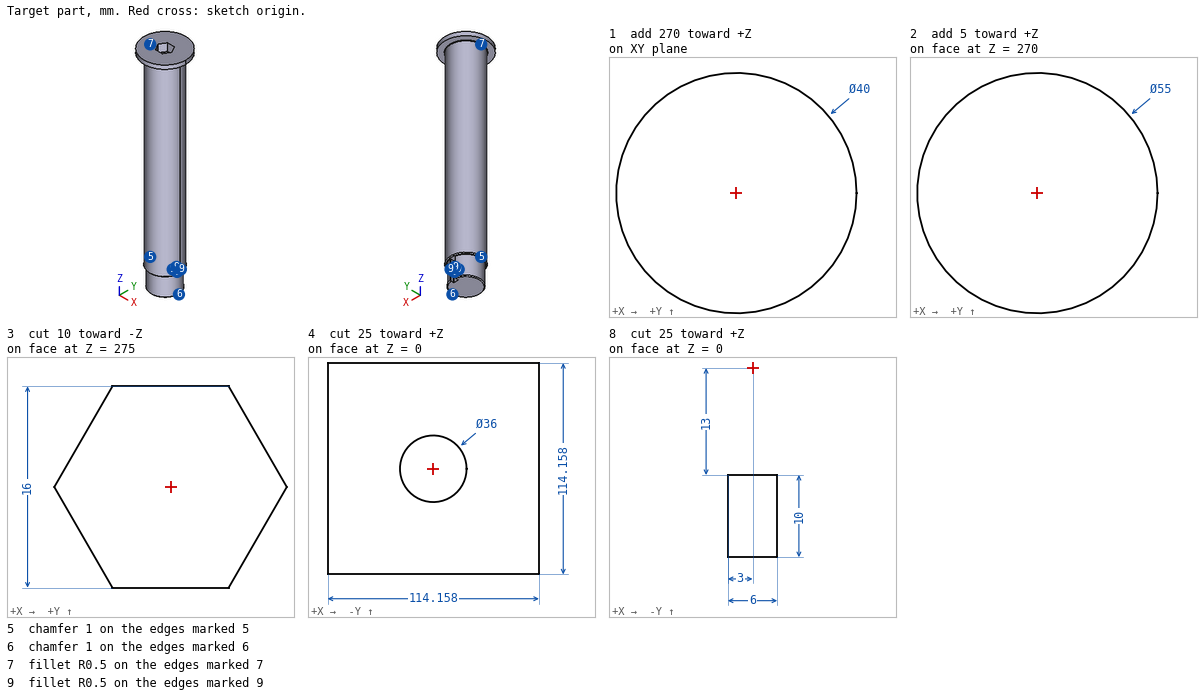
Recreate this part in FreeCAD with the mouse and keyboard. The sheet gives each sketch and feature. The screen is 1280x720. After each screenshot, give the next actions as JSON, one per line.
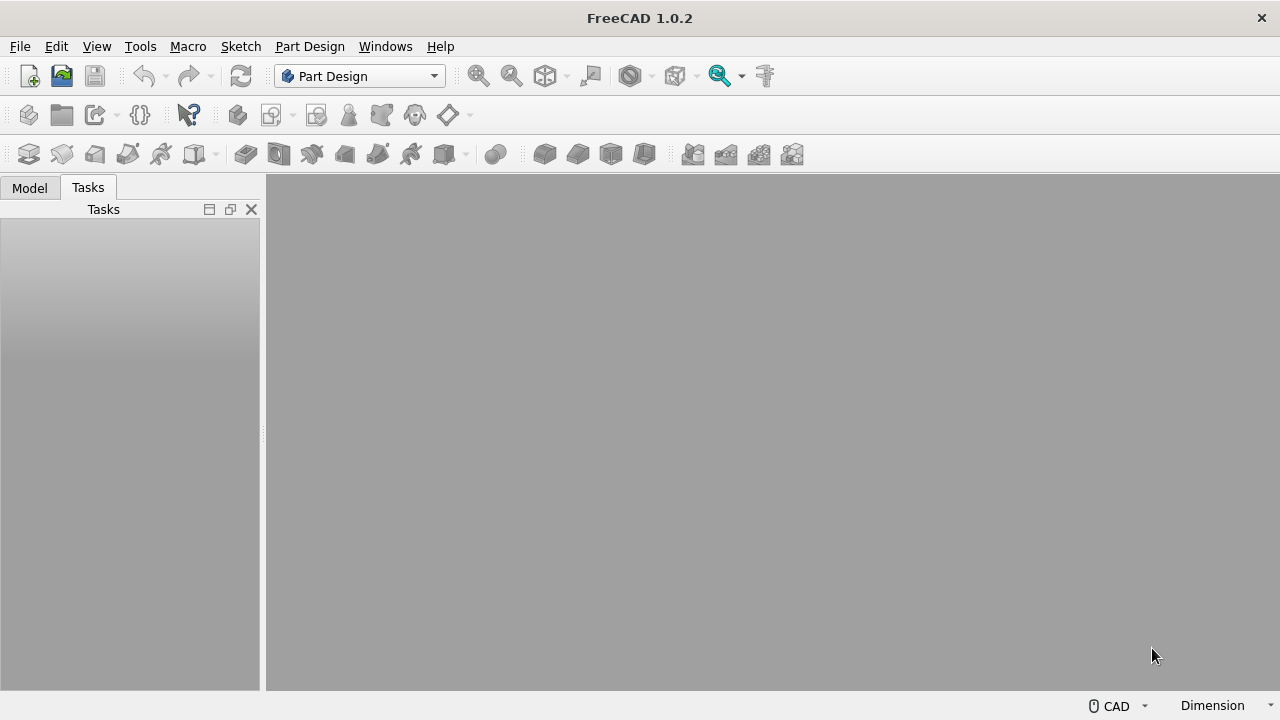
{"action": "left_click", "coordinate": [29, 76]}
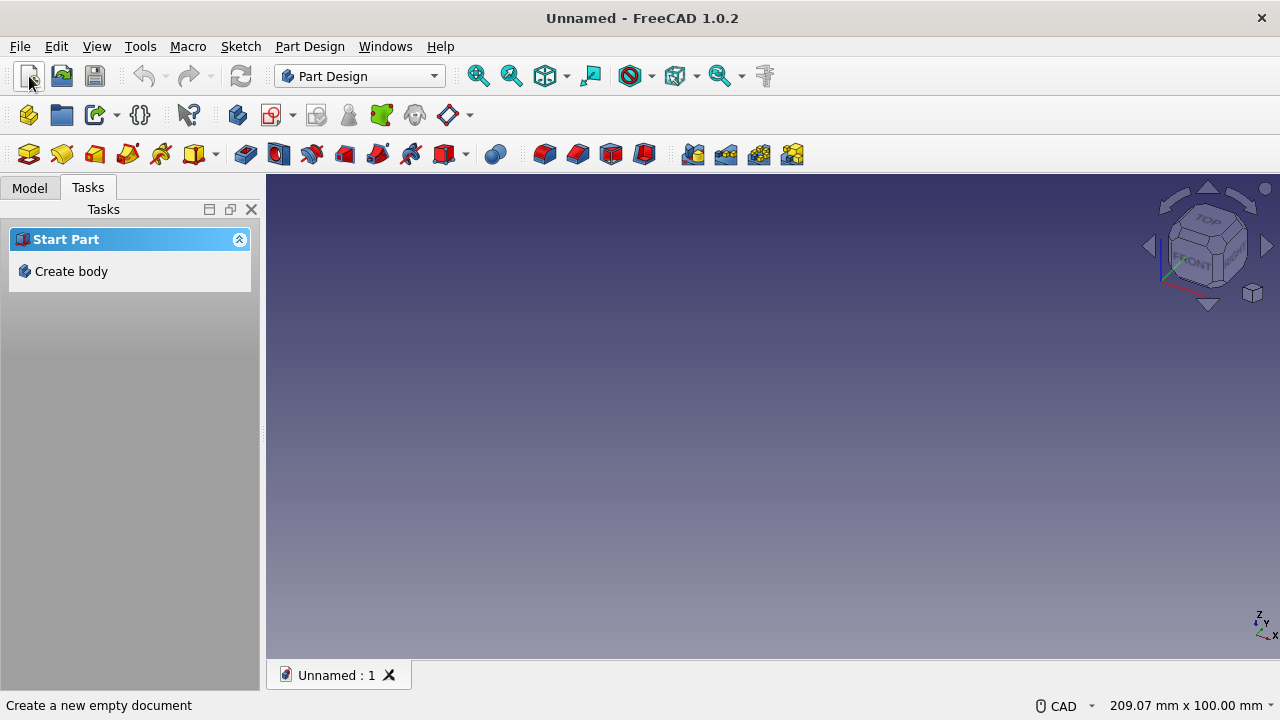
{"action": "left_click", "coordinate": [270, 116]}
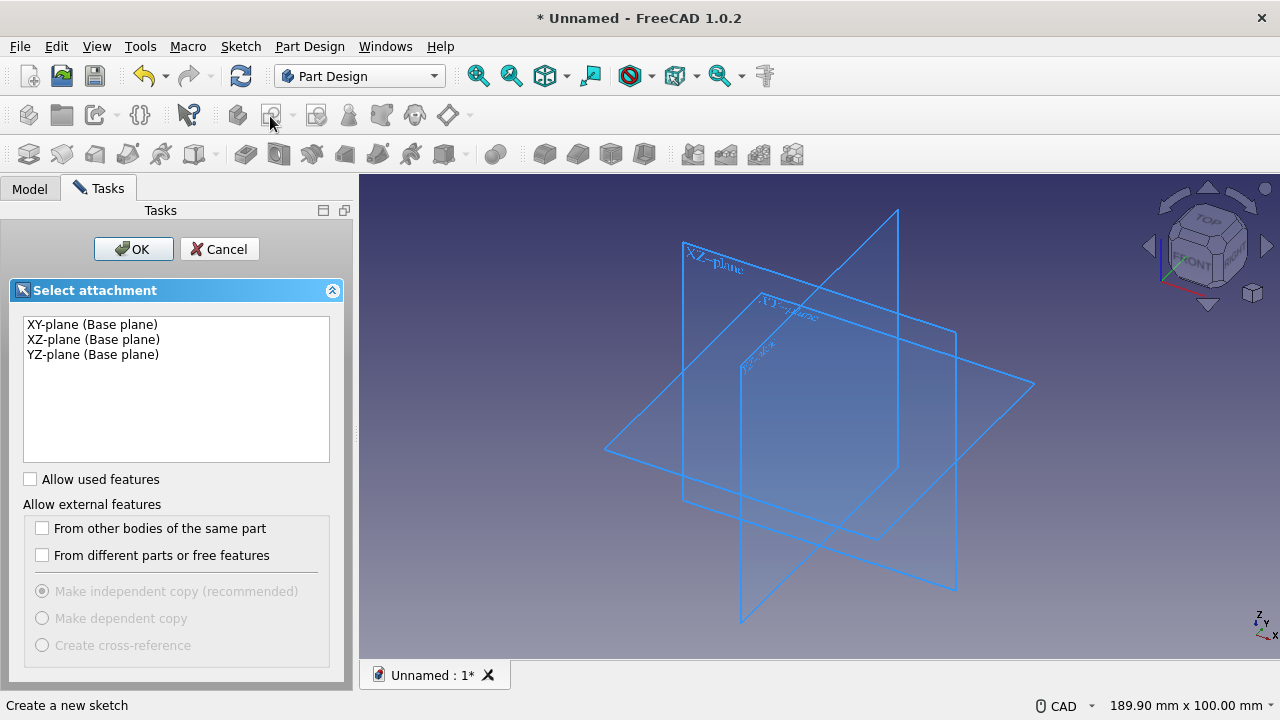
{"action": "left_click", "coordinate": [84, 324]}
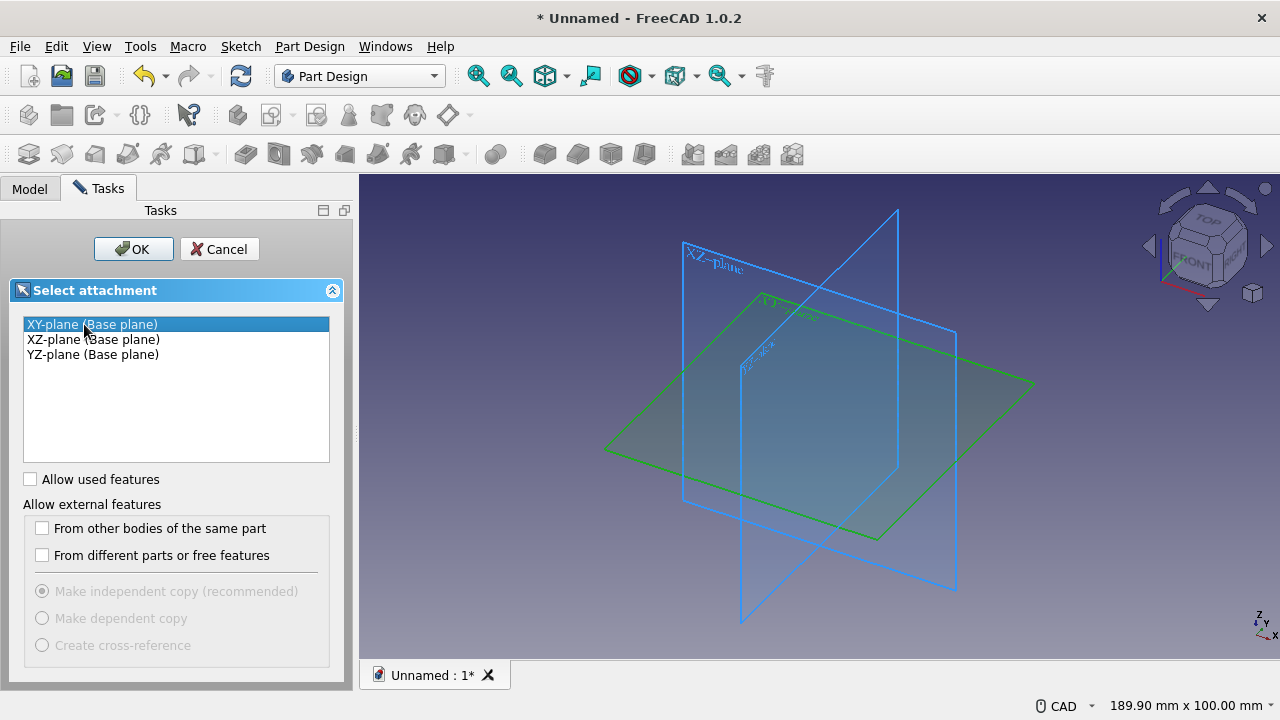
{"action": "left_click", "coordinate": [134, 249]}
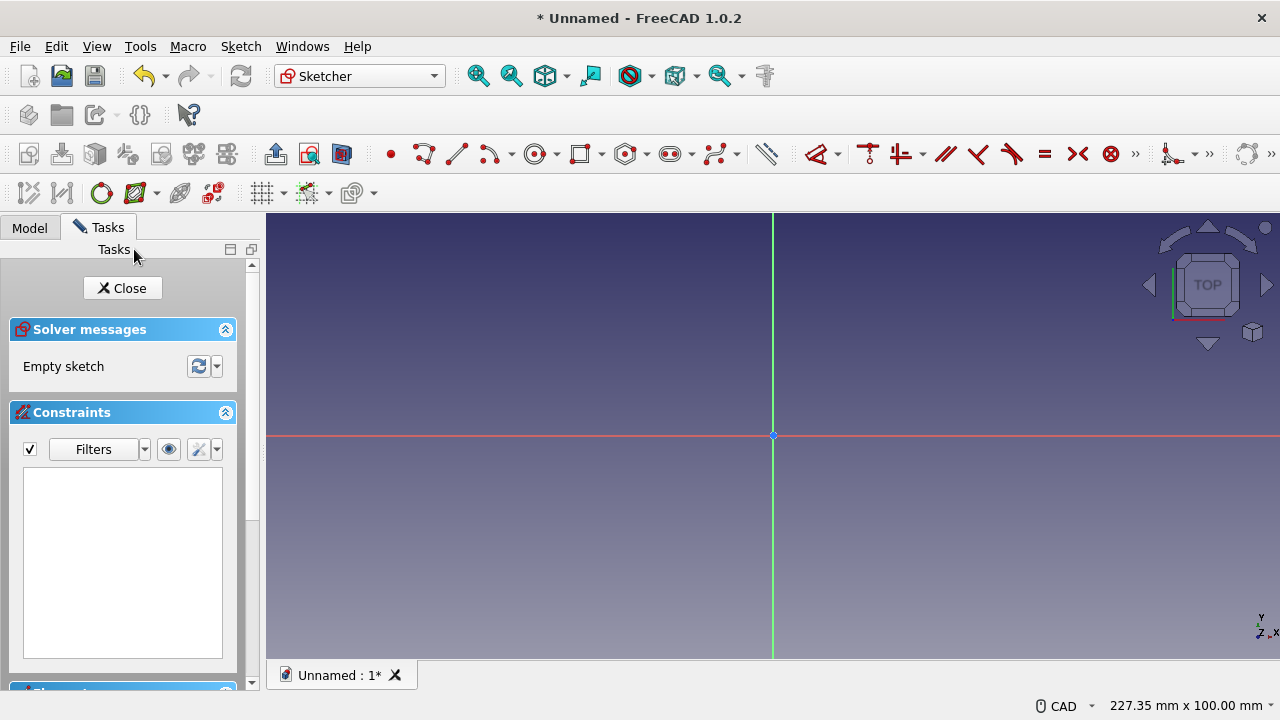
{"action": "scroll", "coordinate": [912, 436], "scroll_direction": "up", "scroll_amount": 2}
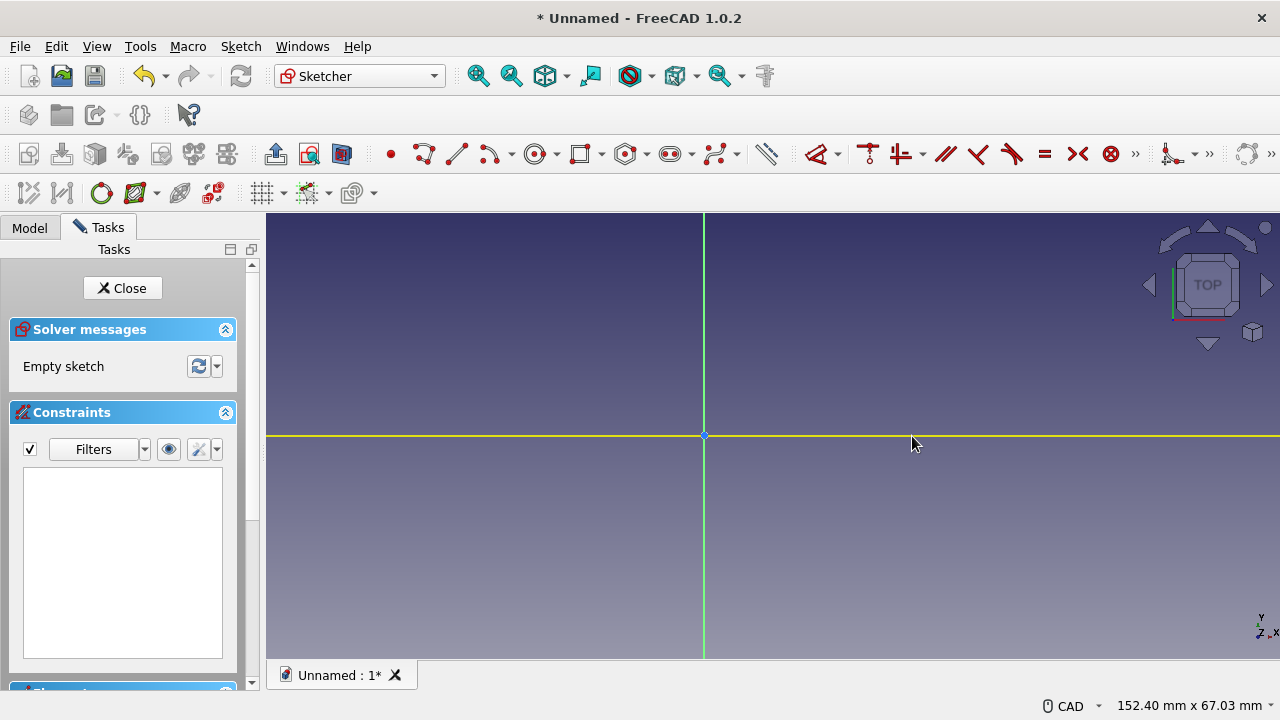
{"action": "left_click", "coordinate": [534, 154]}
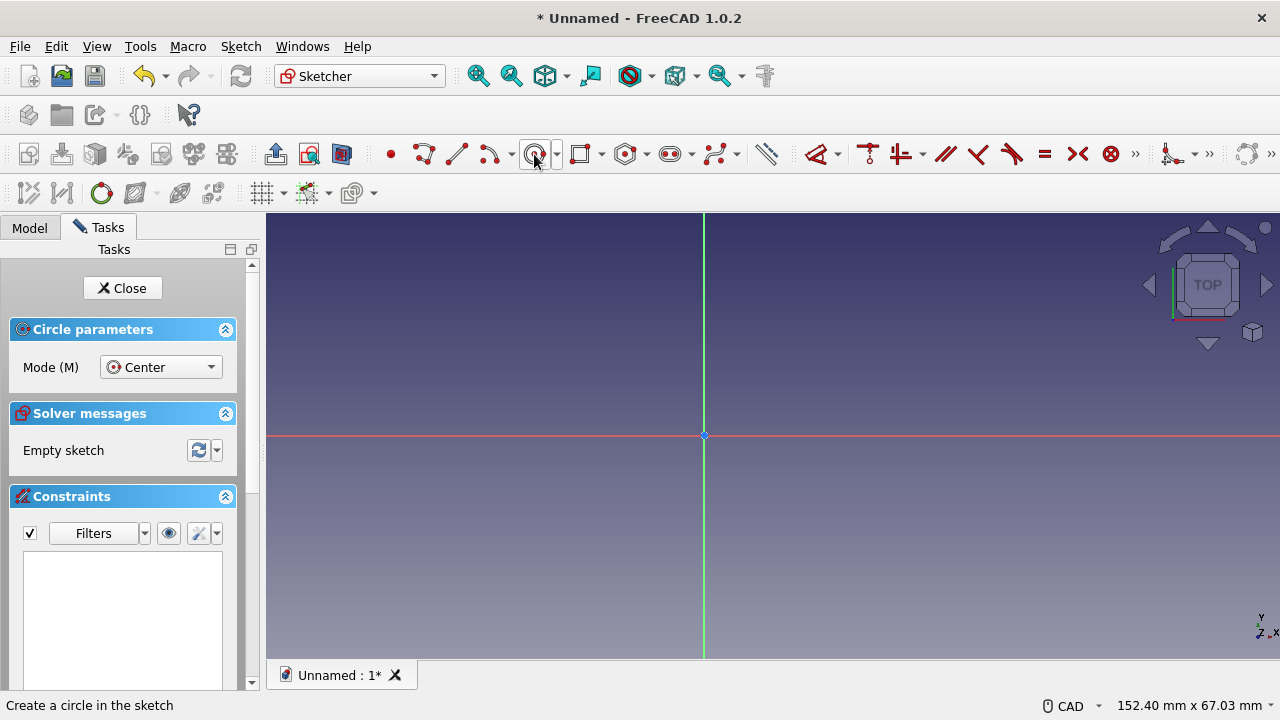
{"action": "left_click", "coordinate": [704, 436]}
{"action": "mouse_move", "coordinate": [798, 342]}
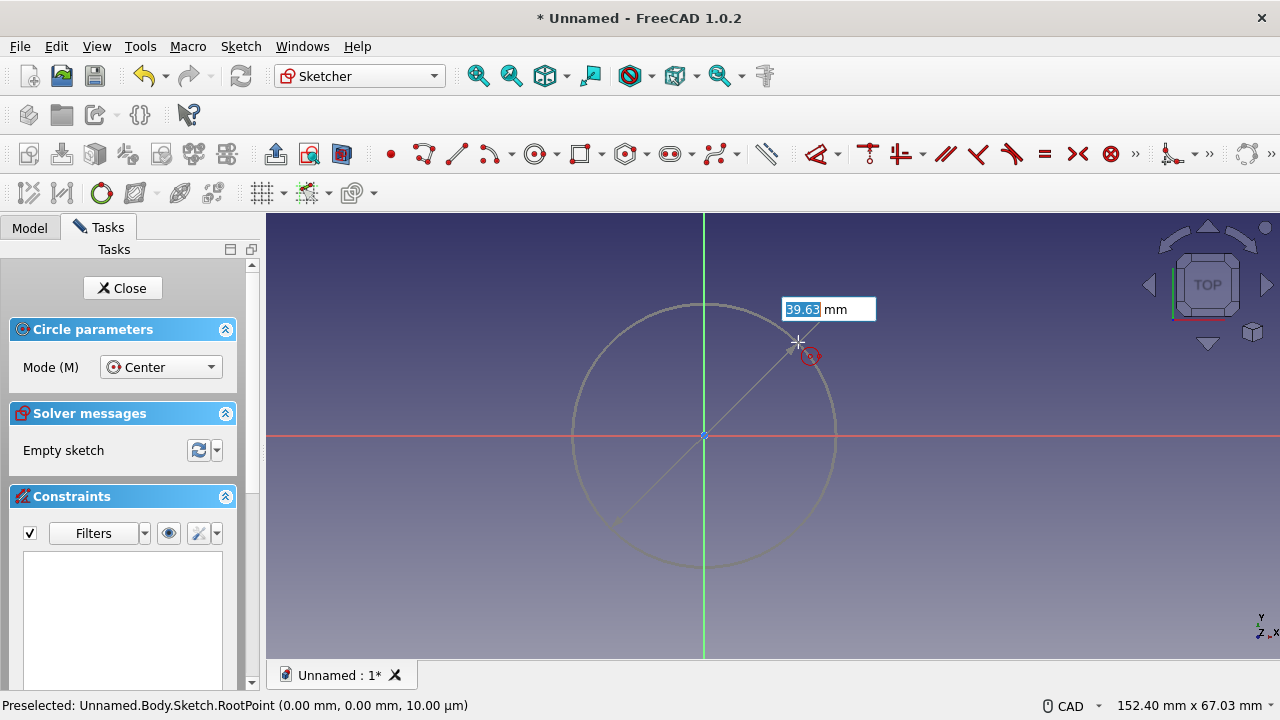
{"action": "type", "text": "40"}
{"action": "key", "text": "Return"}
{"action": "key", "text": "Escape"}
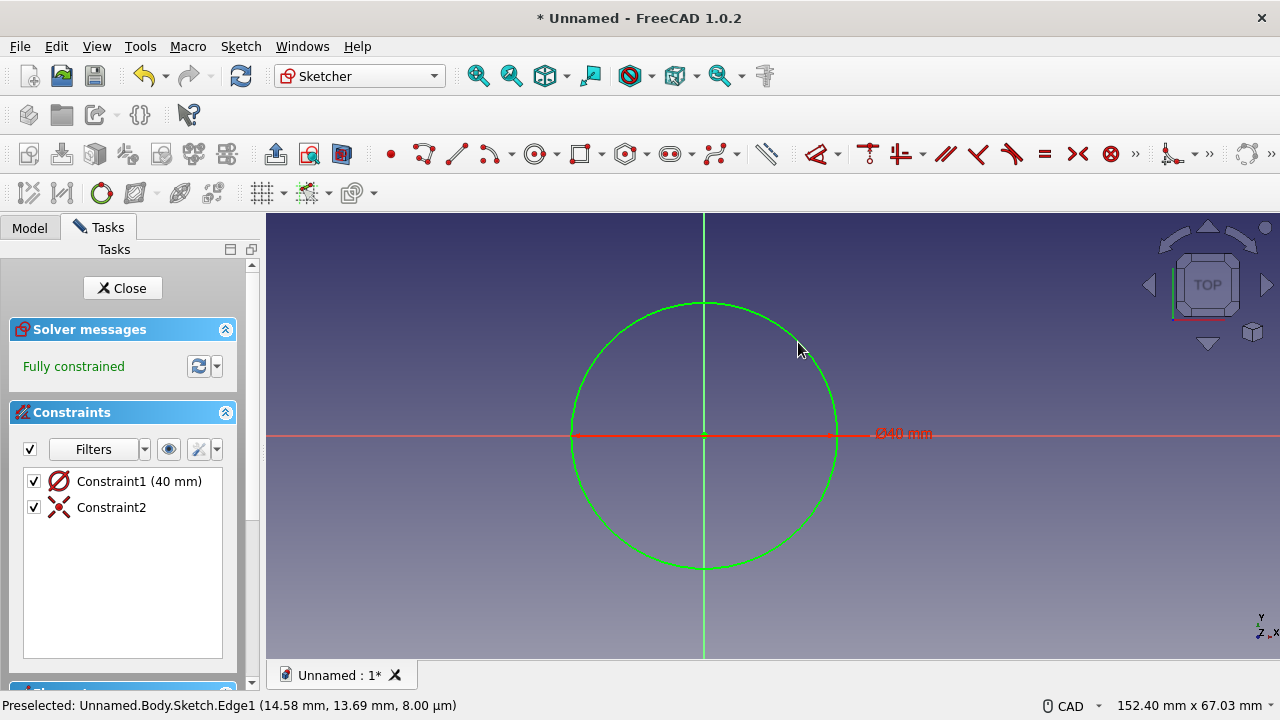
{"action": "left_click", "coordinate": [123, 288]}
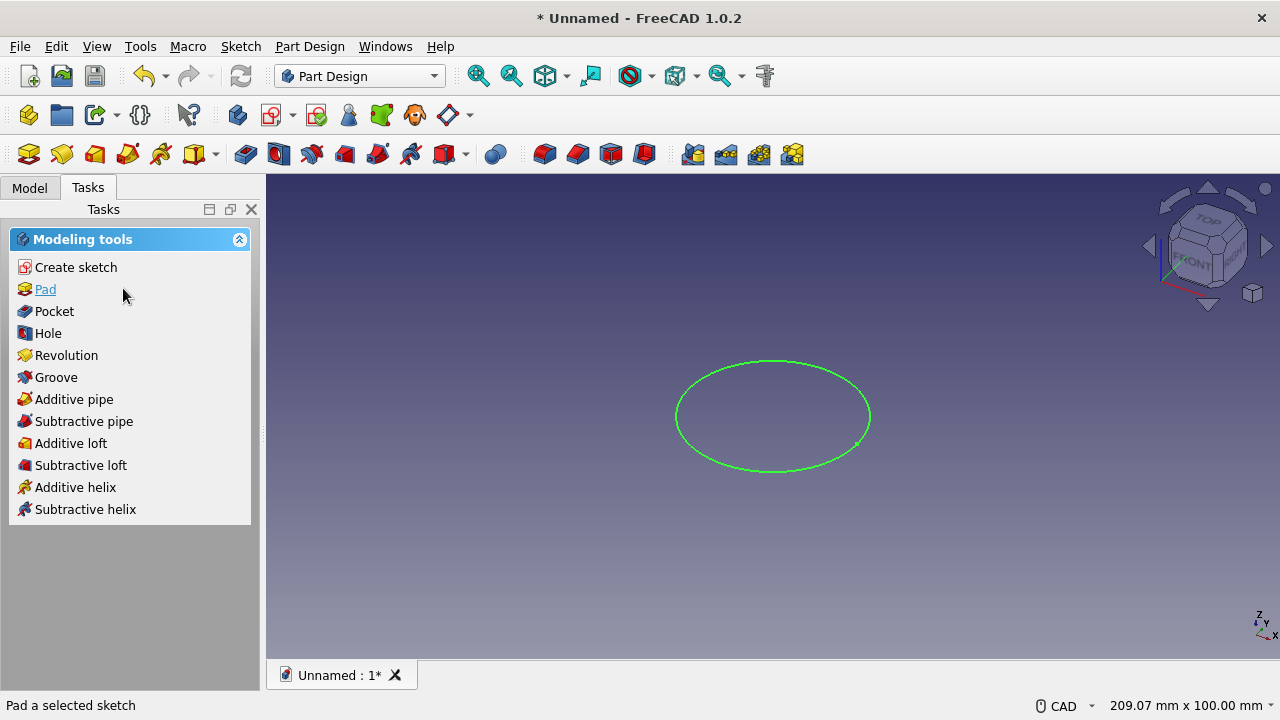
{"action": "left_click", "coordinate": [29, 154]}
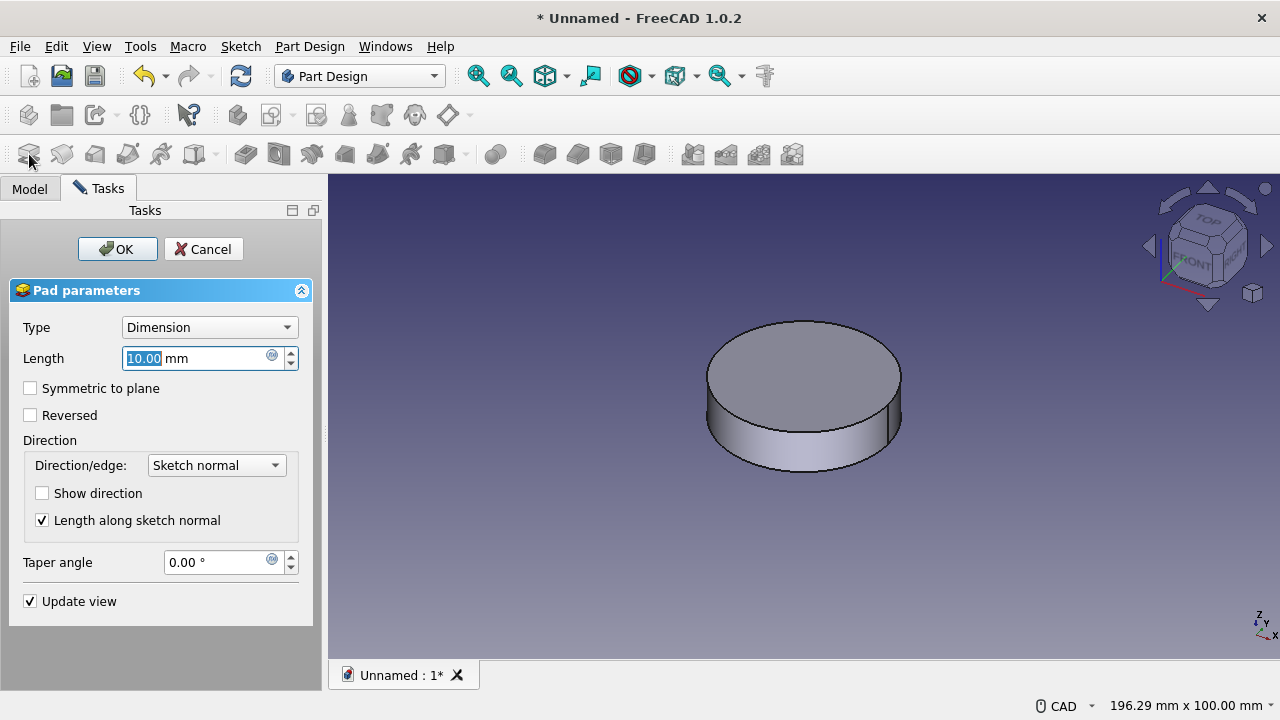
{"action": "type", "text": "270"}
{"action": "key", "text": "Tab"}